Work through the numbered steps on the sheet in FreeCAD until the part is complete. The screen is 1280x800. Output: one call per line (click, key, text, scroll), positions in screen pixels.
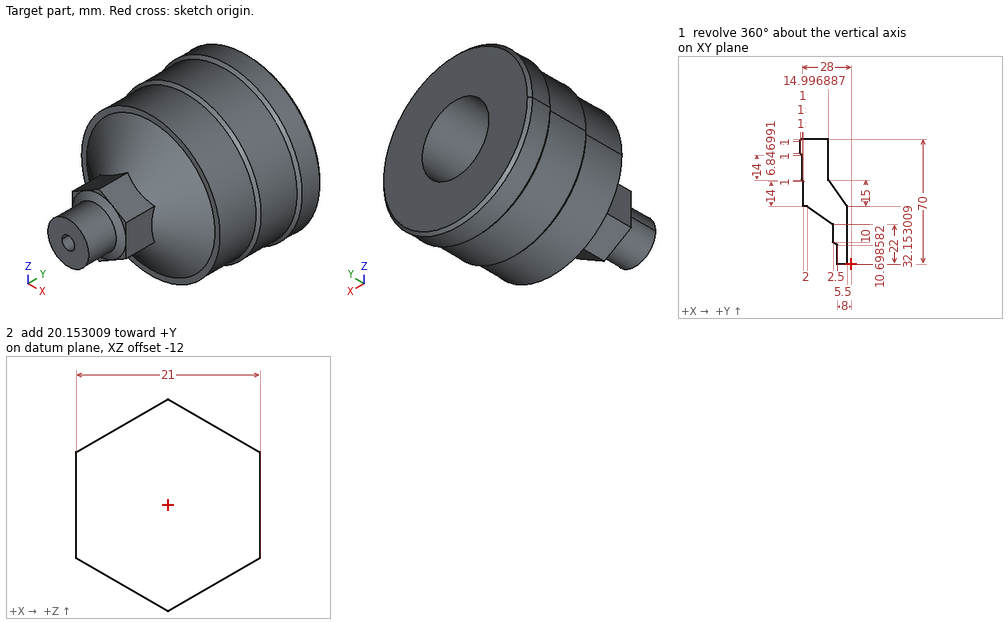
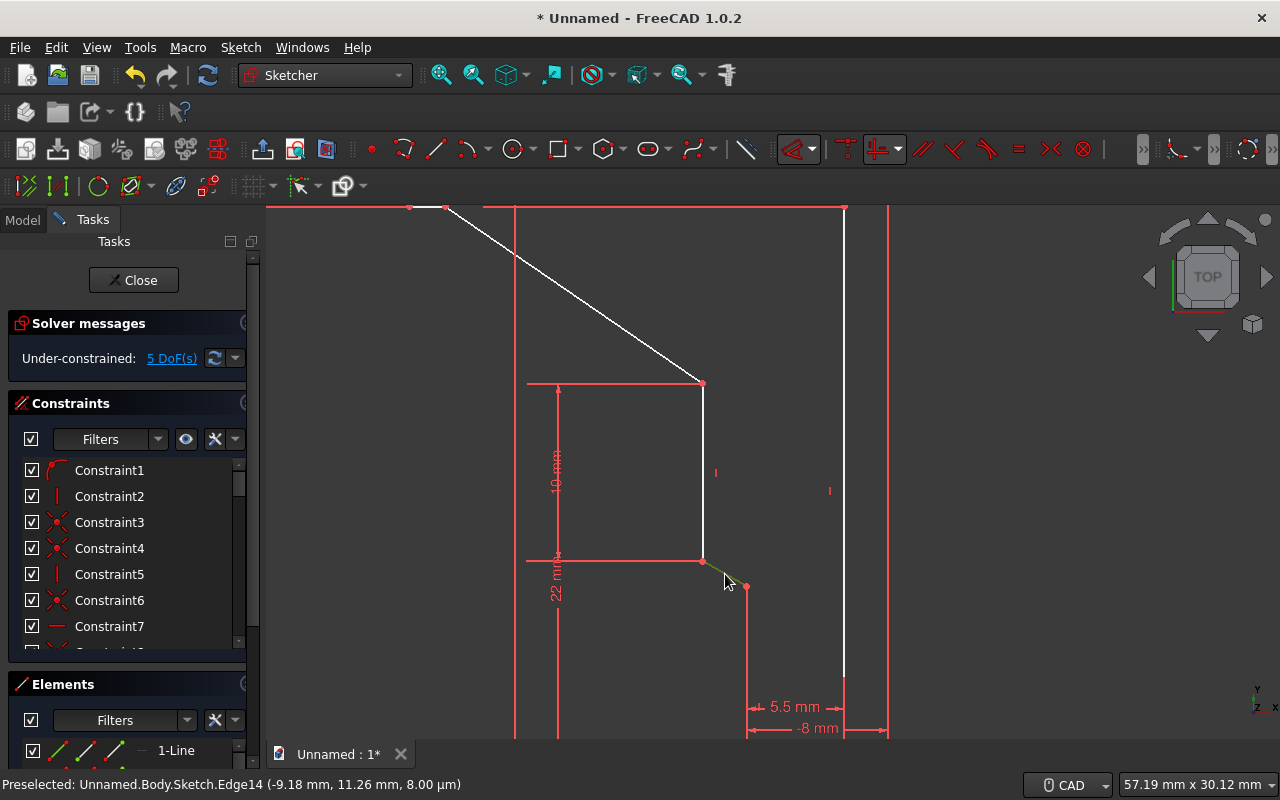
click(814, 150)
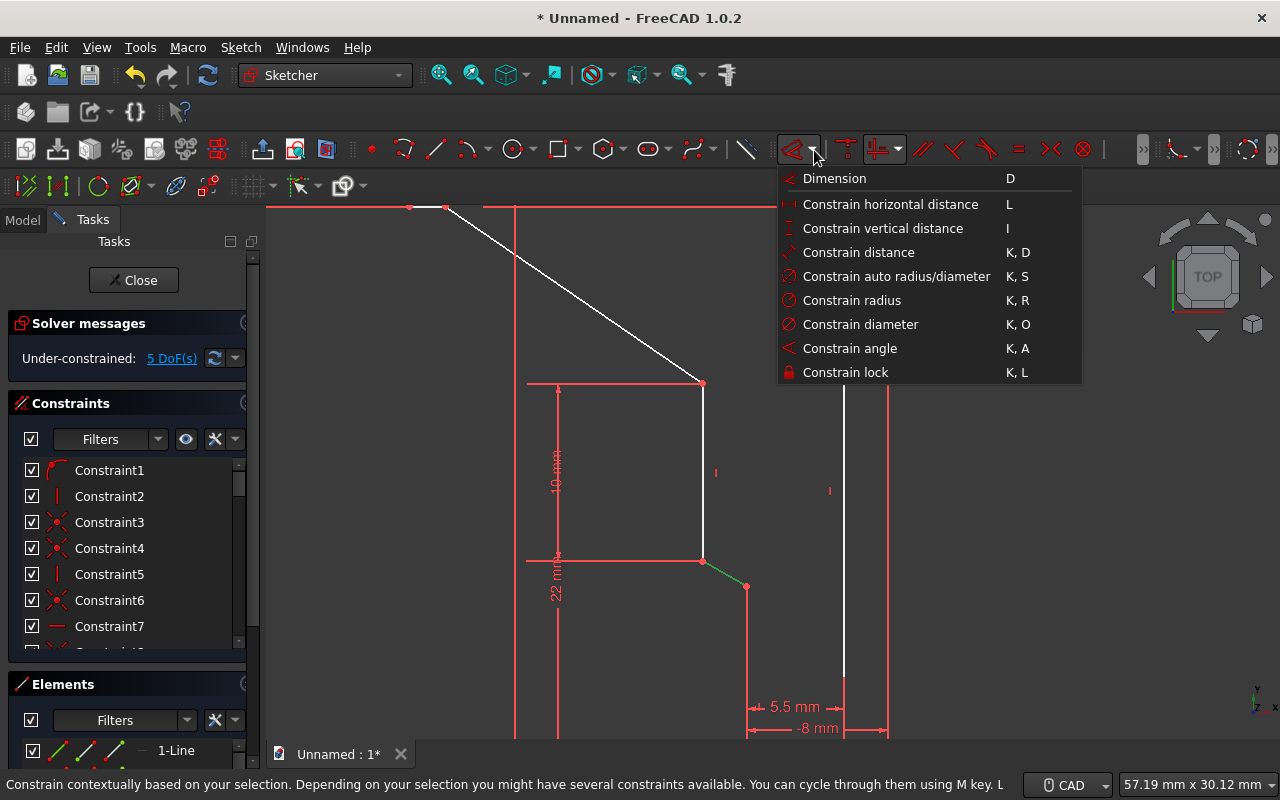
click(930, 204)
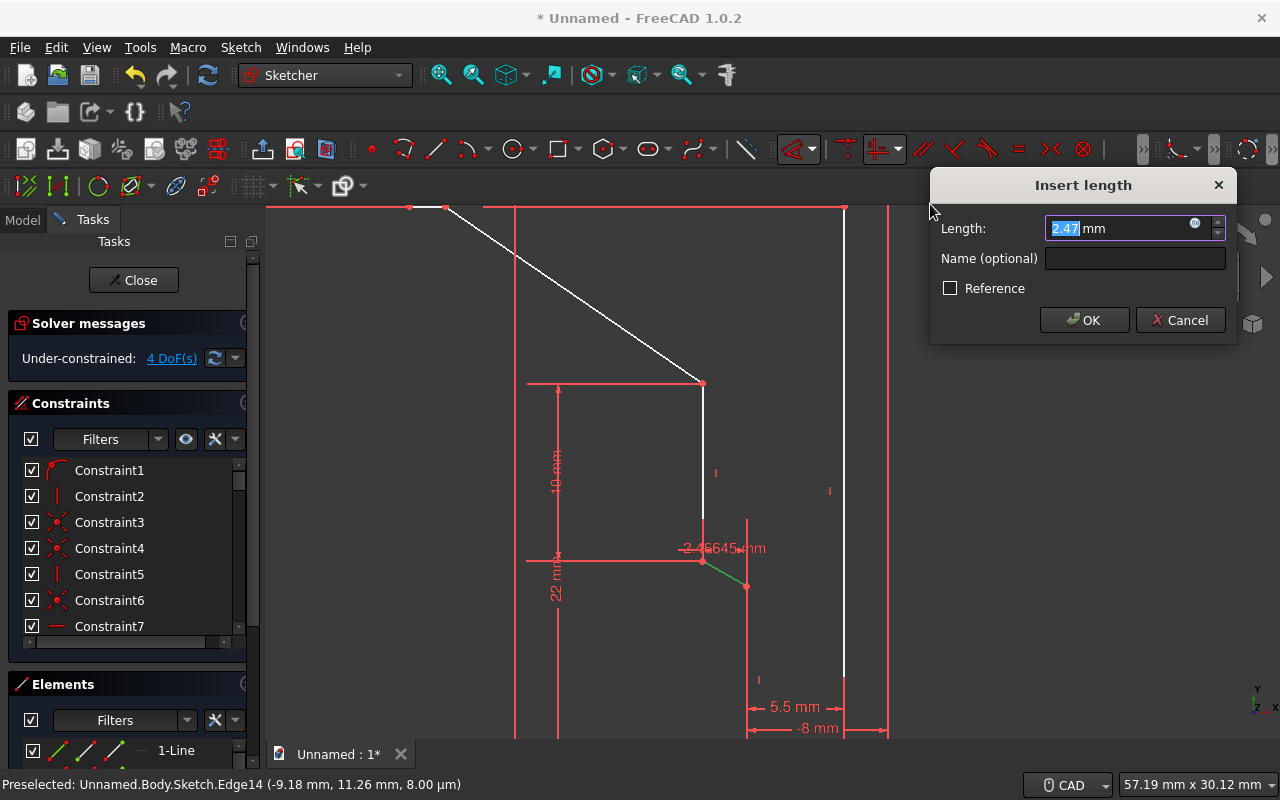
text(2.5)
key(Return)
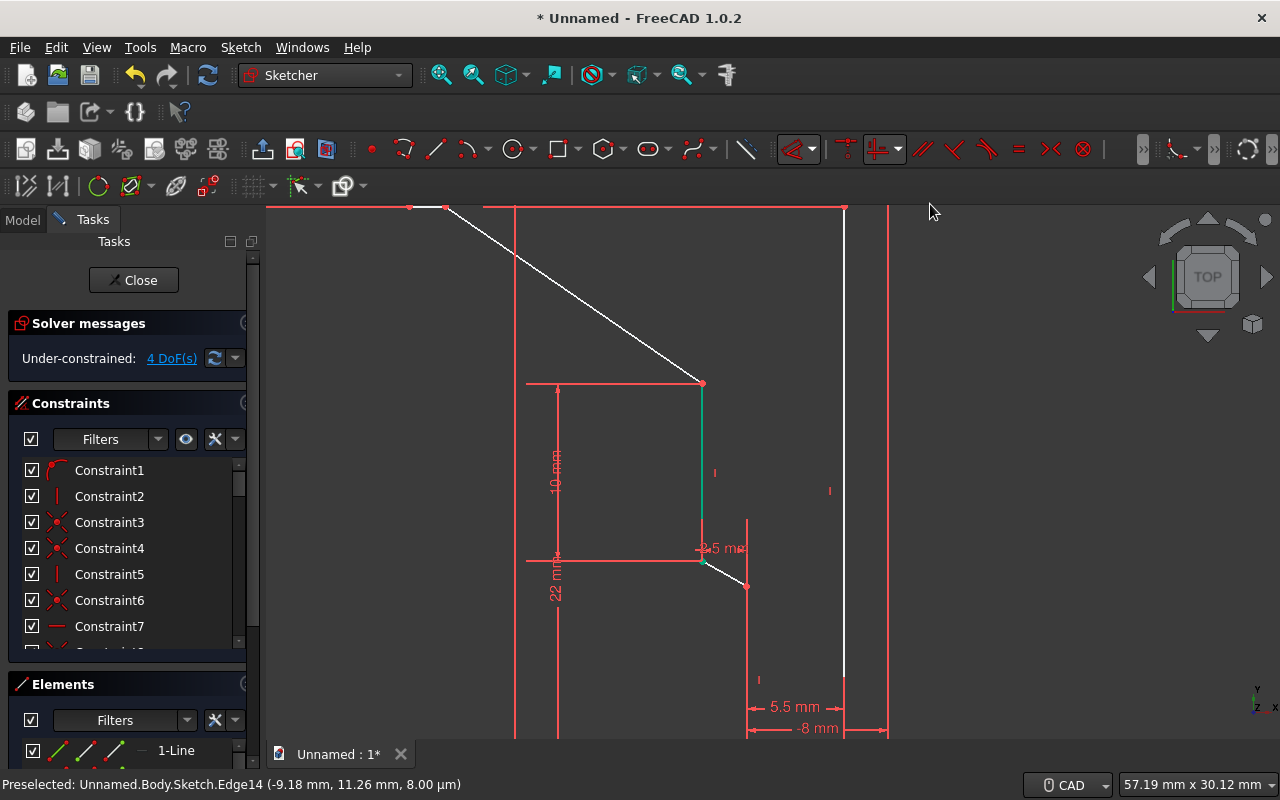
scroll(728, 576, down, 7)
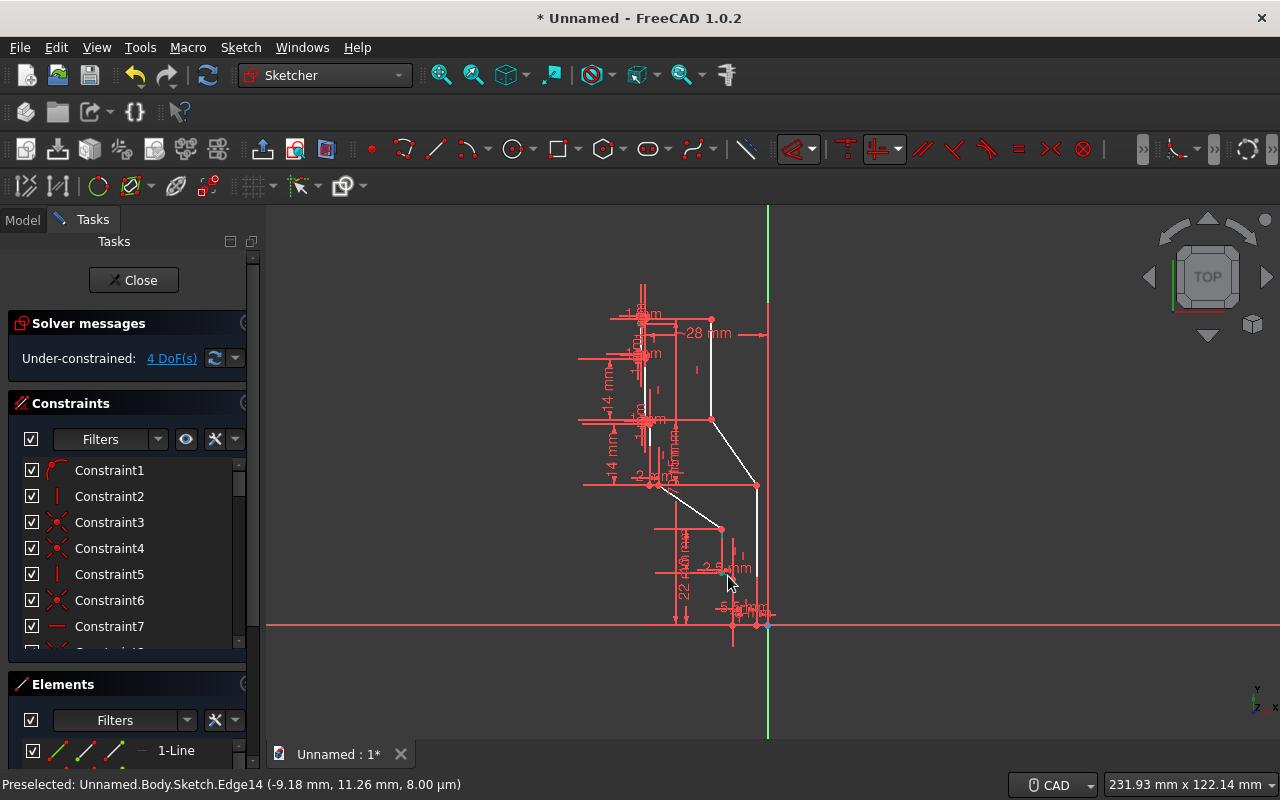
scroll(641, 333, up, 3)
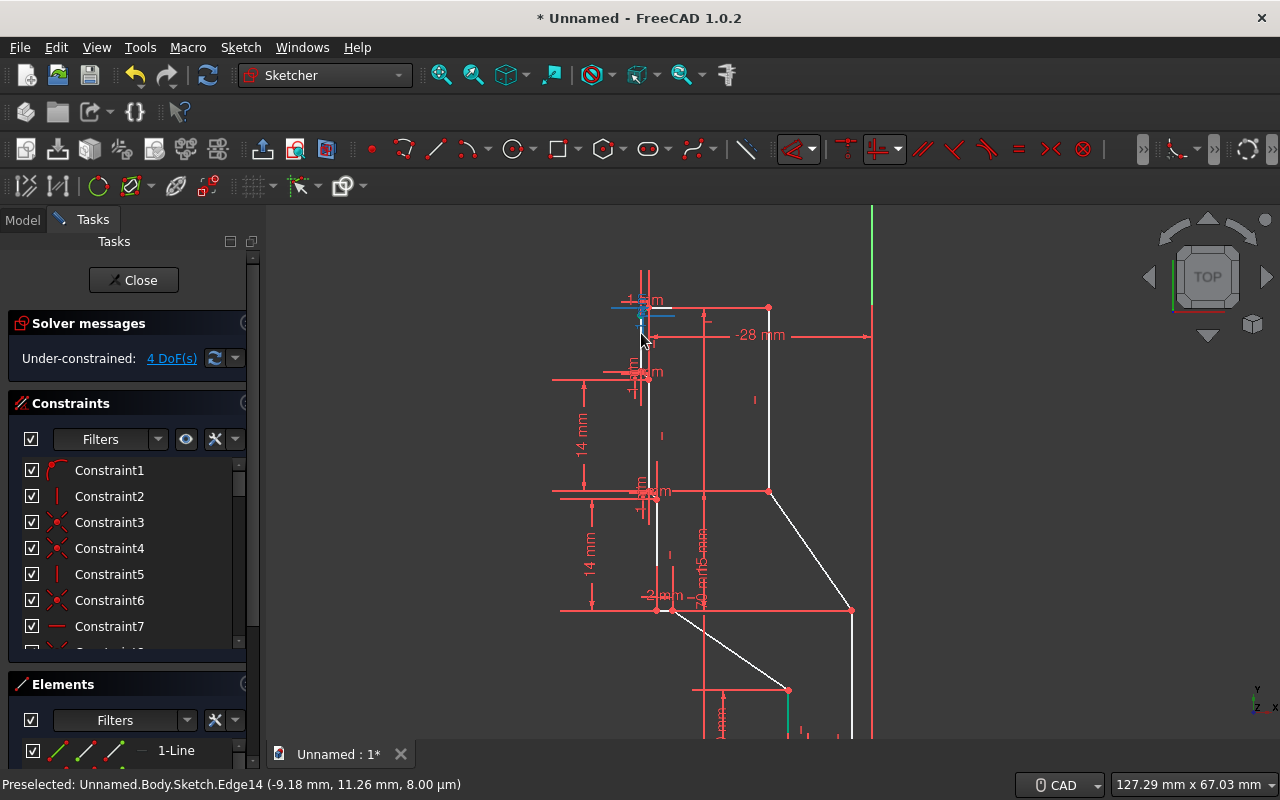
click(641, 332)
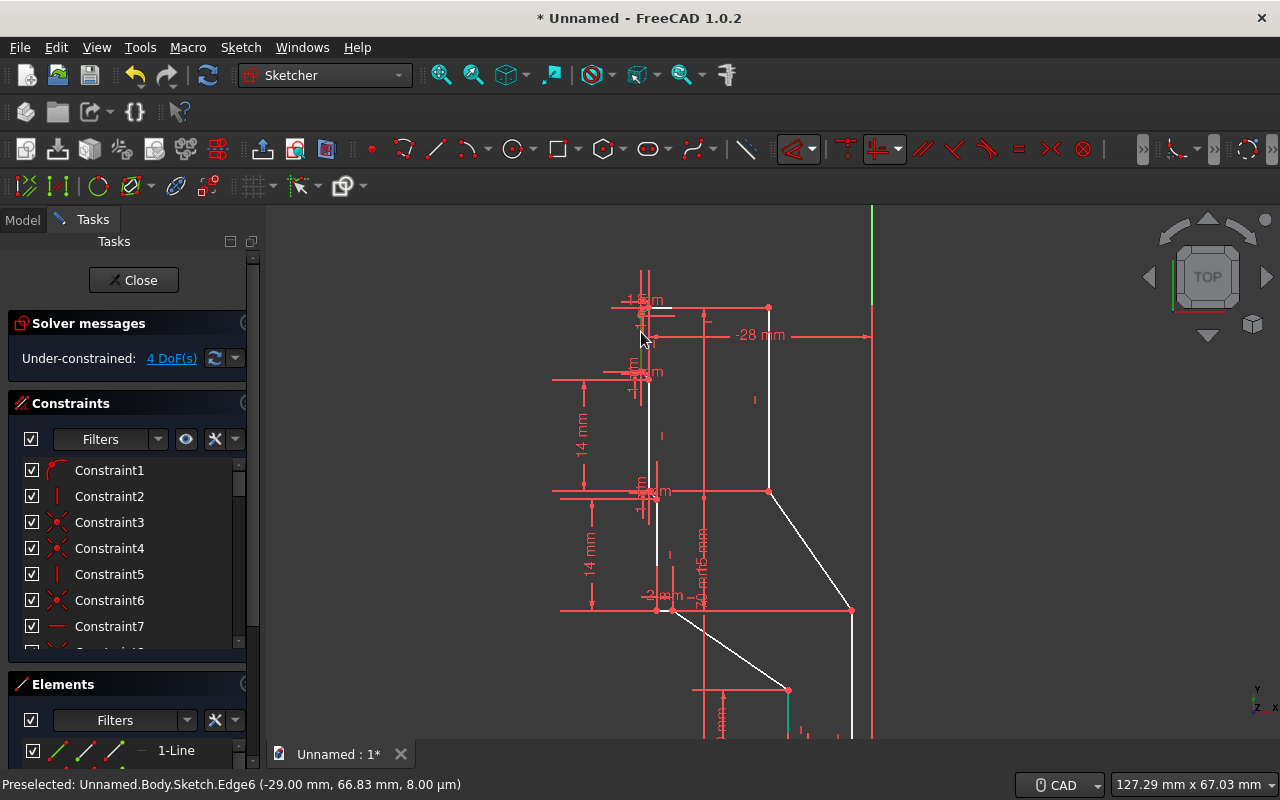
click(814, 150)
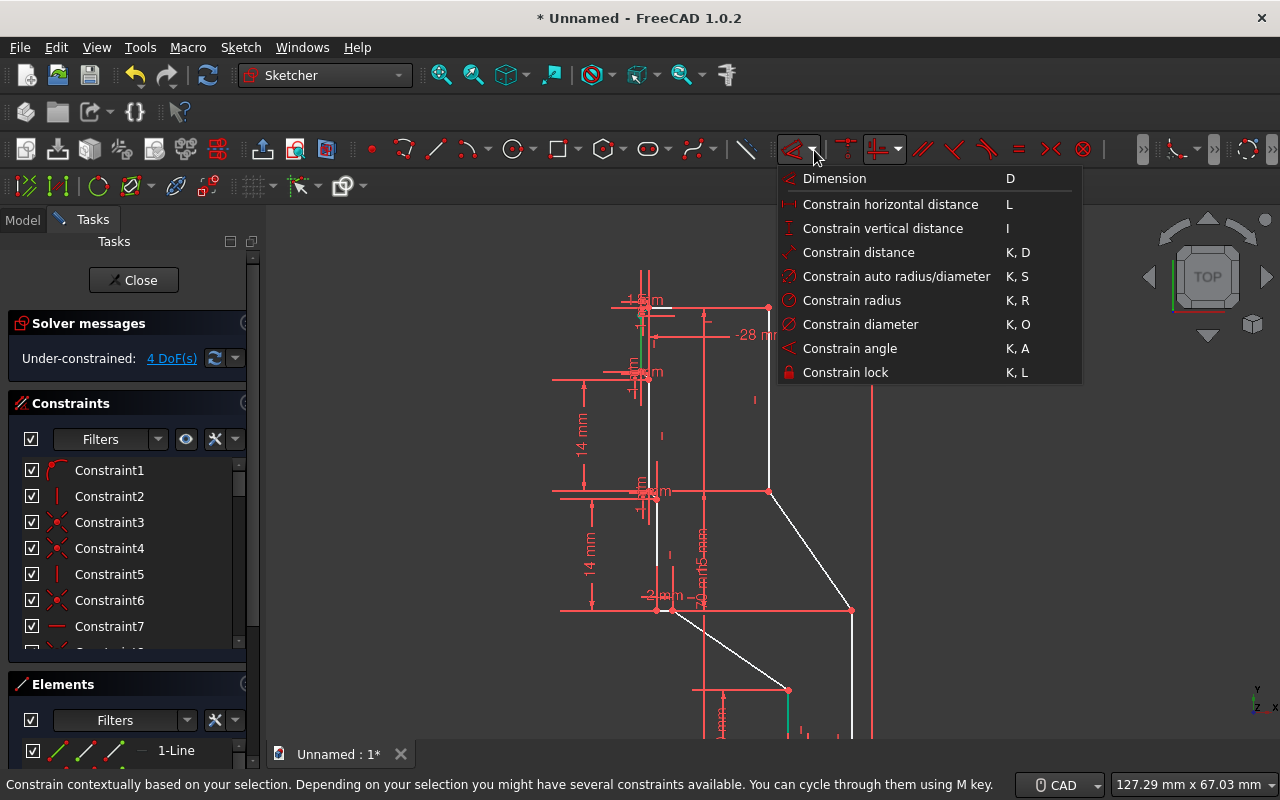
click(930, 228)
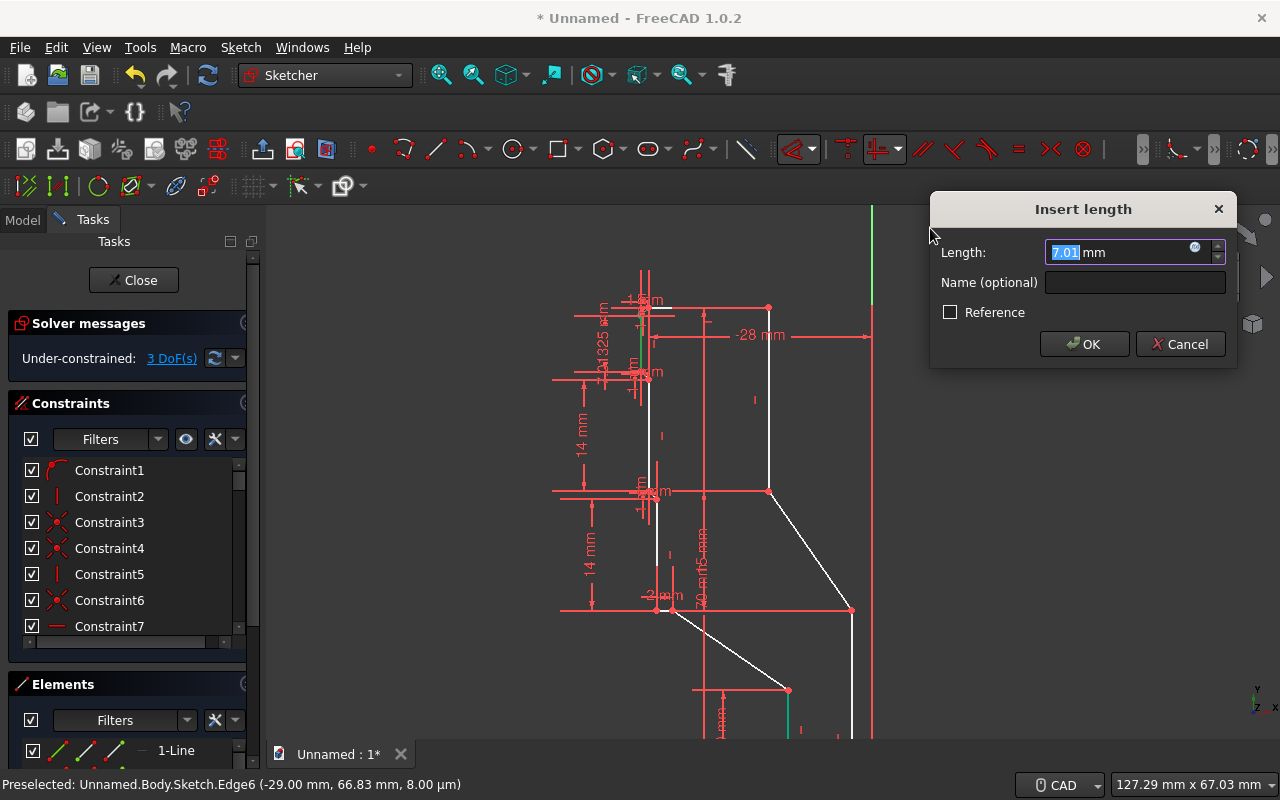
text(6.846991)
key(Return)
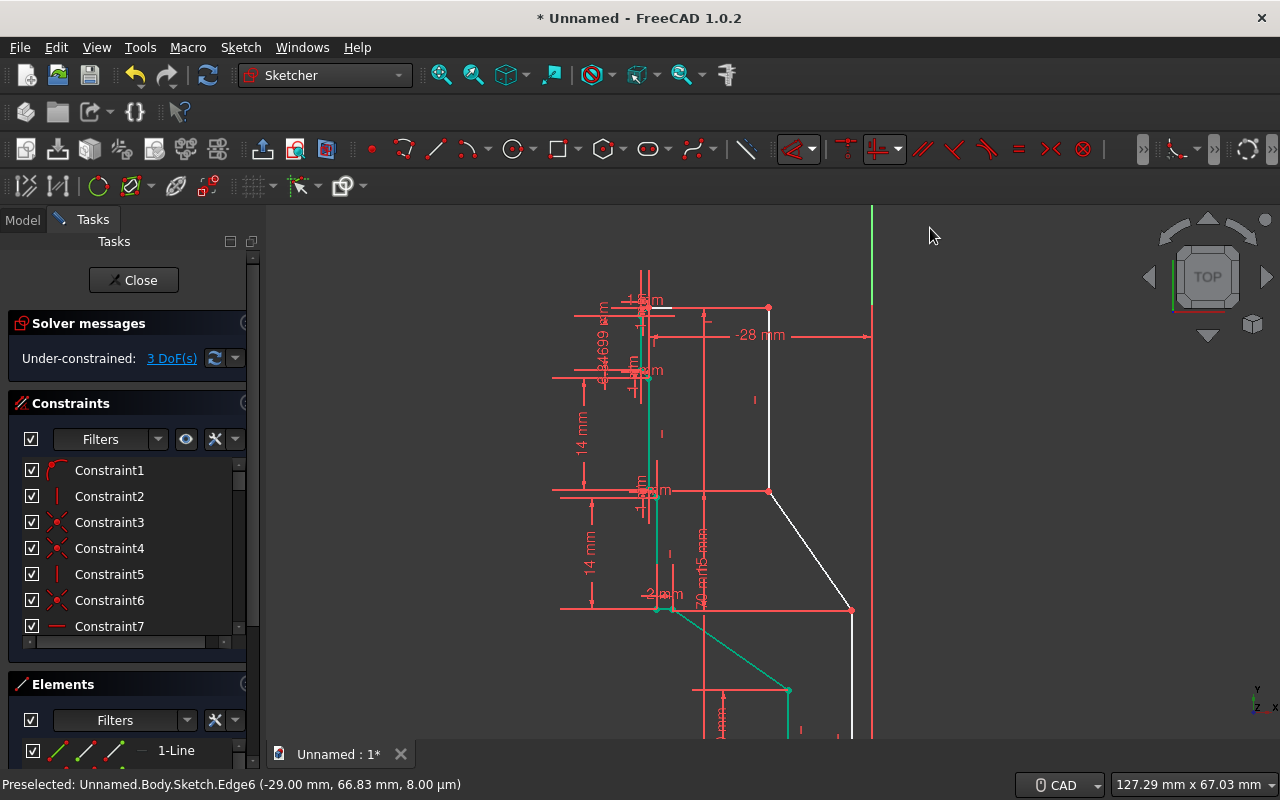
click(852, 687)